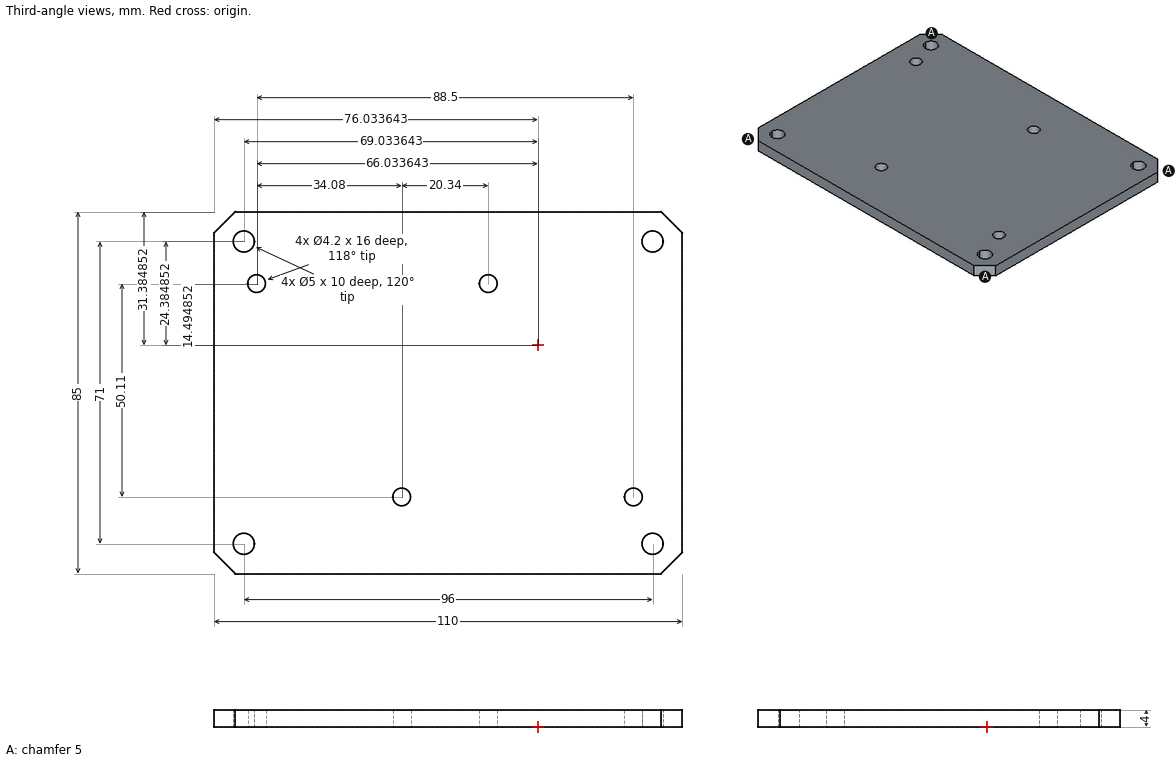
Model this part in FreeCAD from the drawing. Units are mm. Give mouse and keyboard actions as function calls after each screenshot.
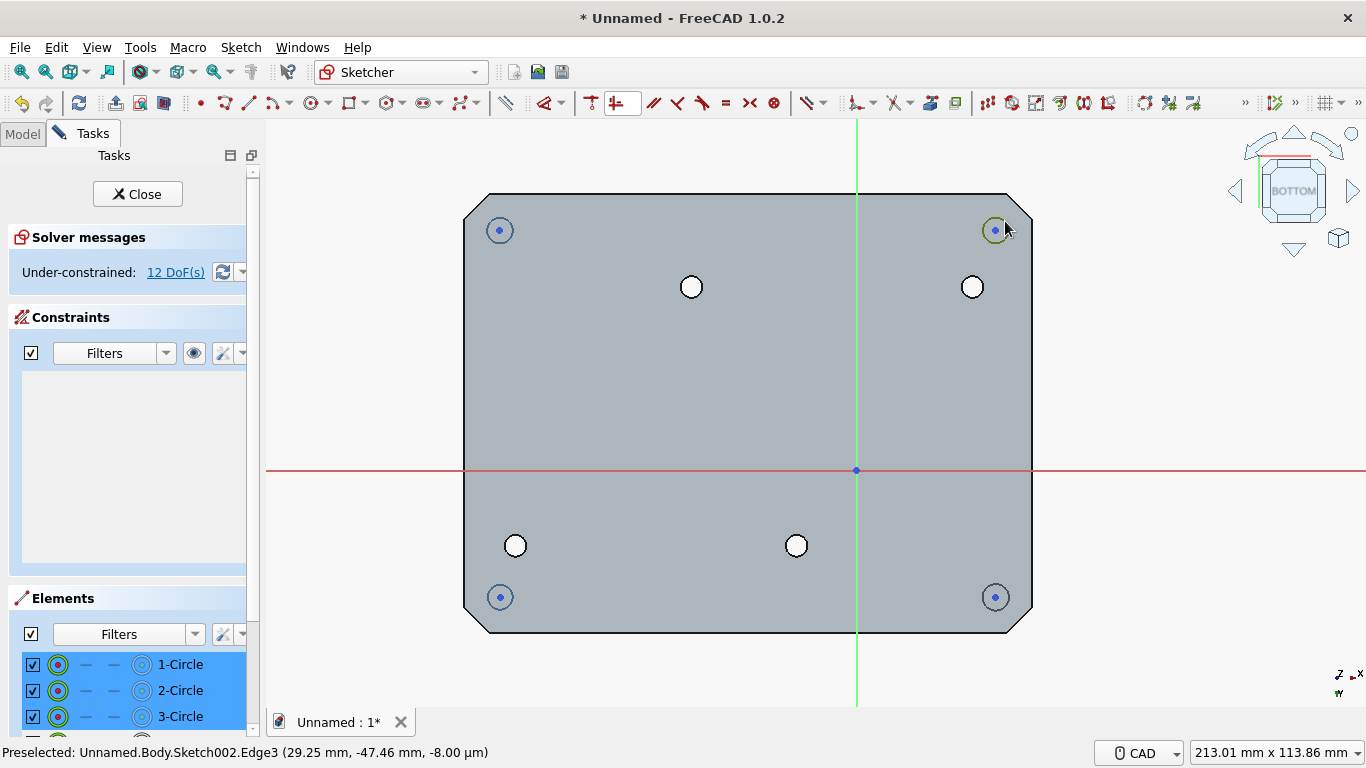
click(1005, 588)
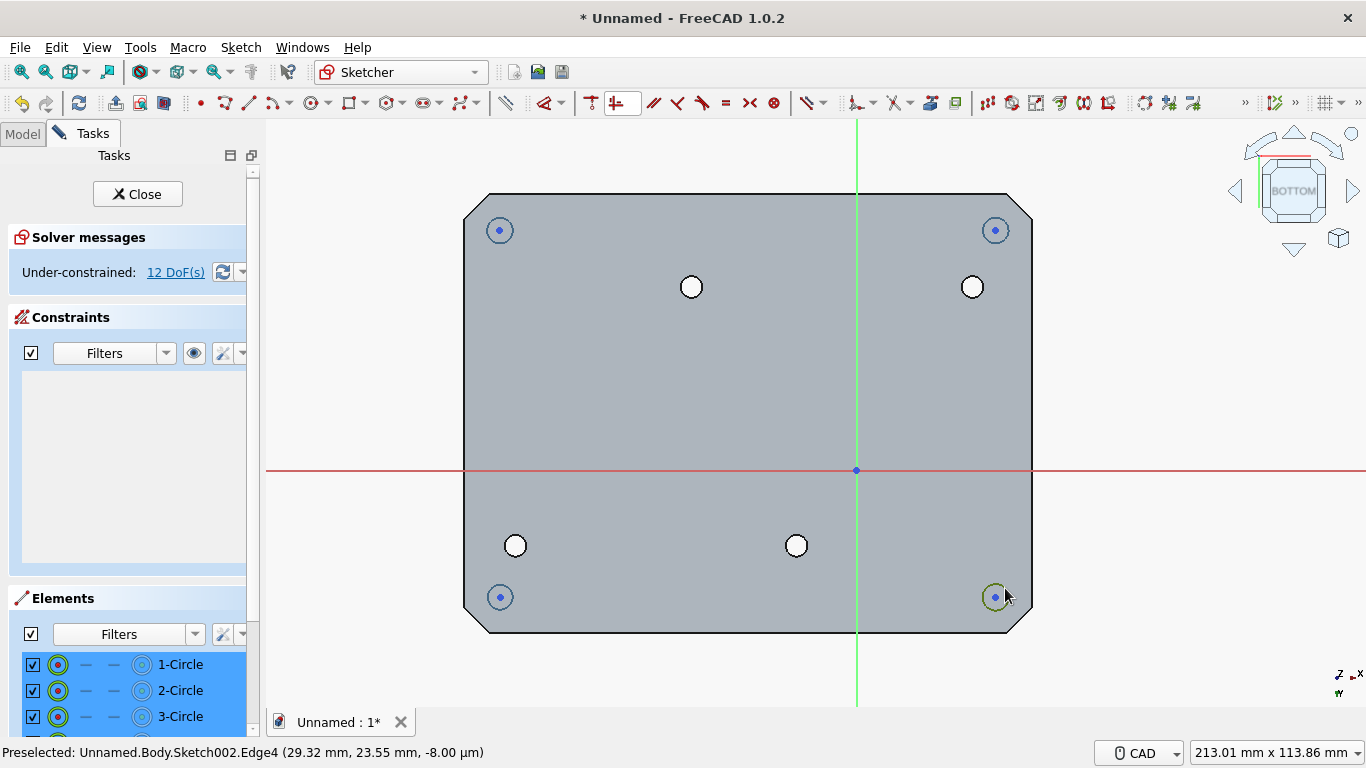
click(726, 104)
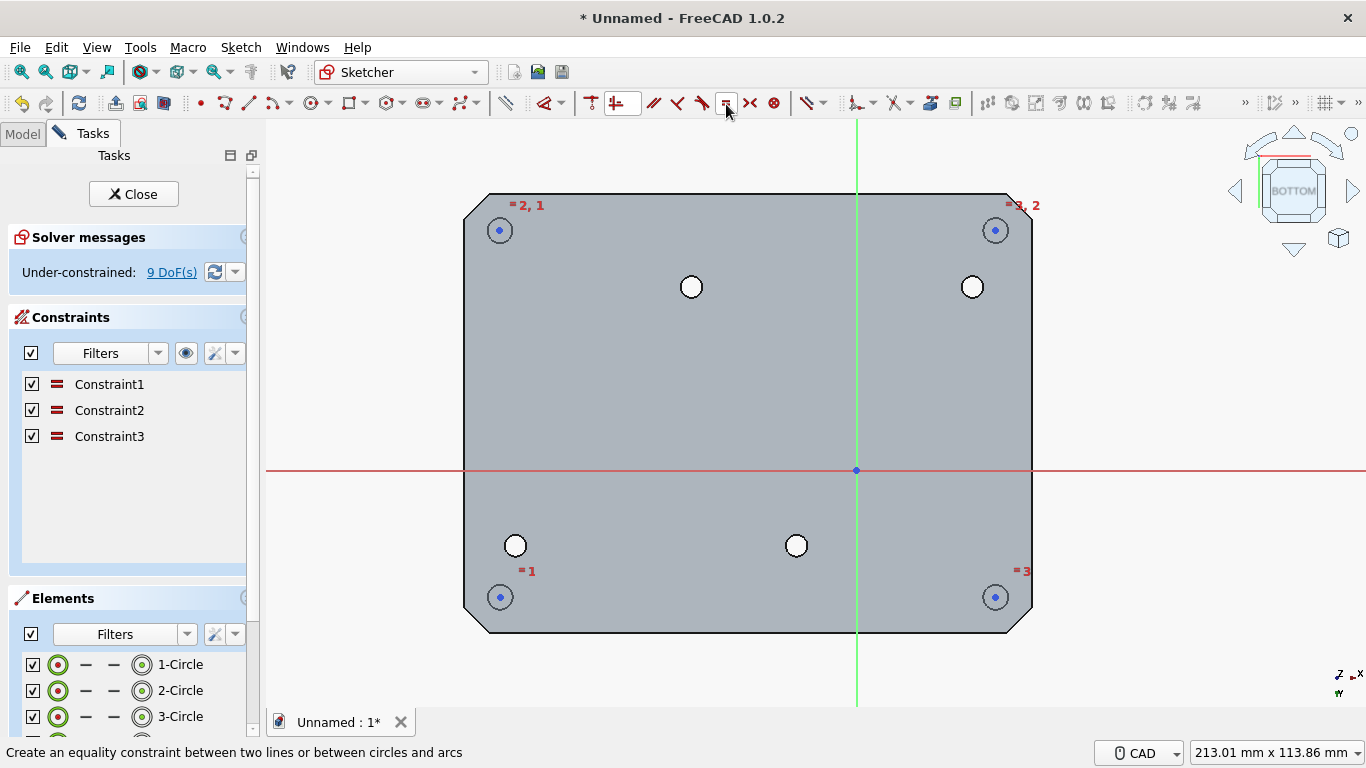
click(500, 597)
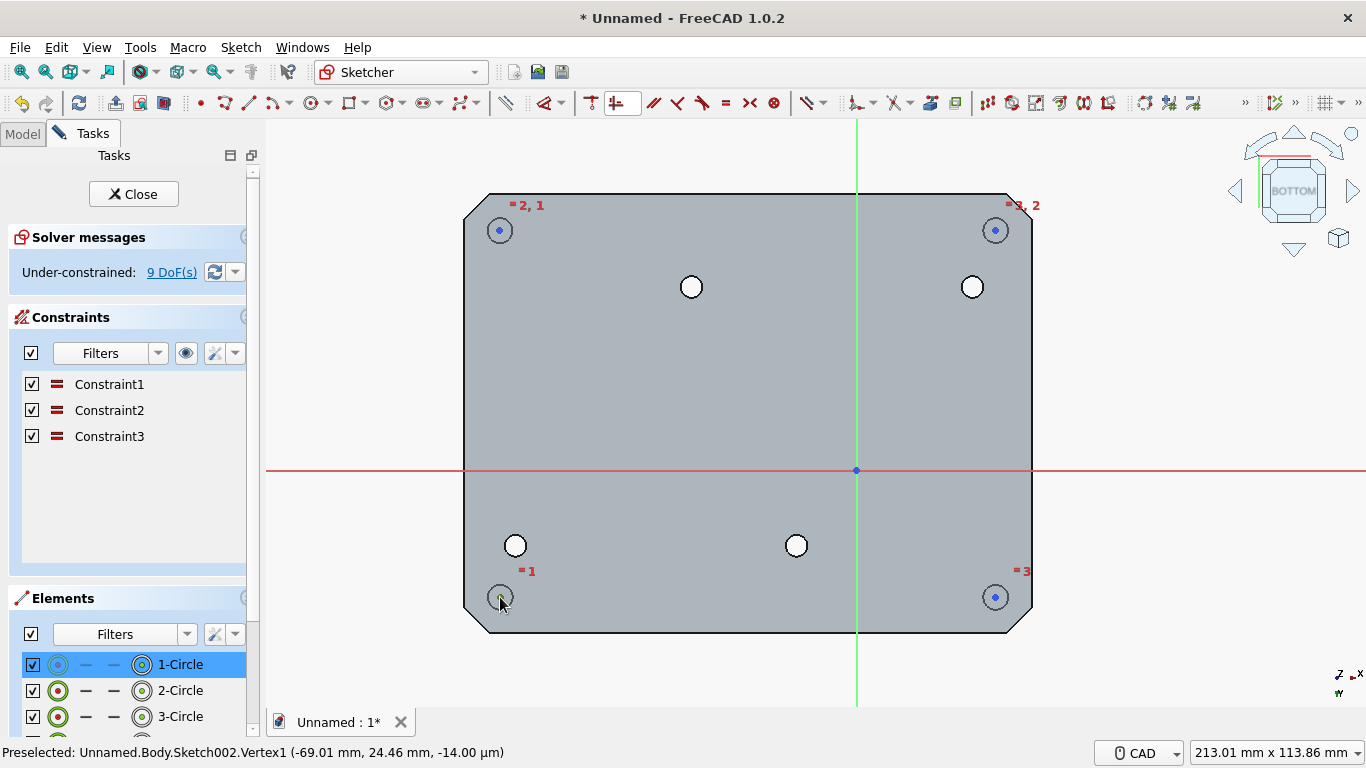
click(500, 231)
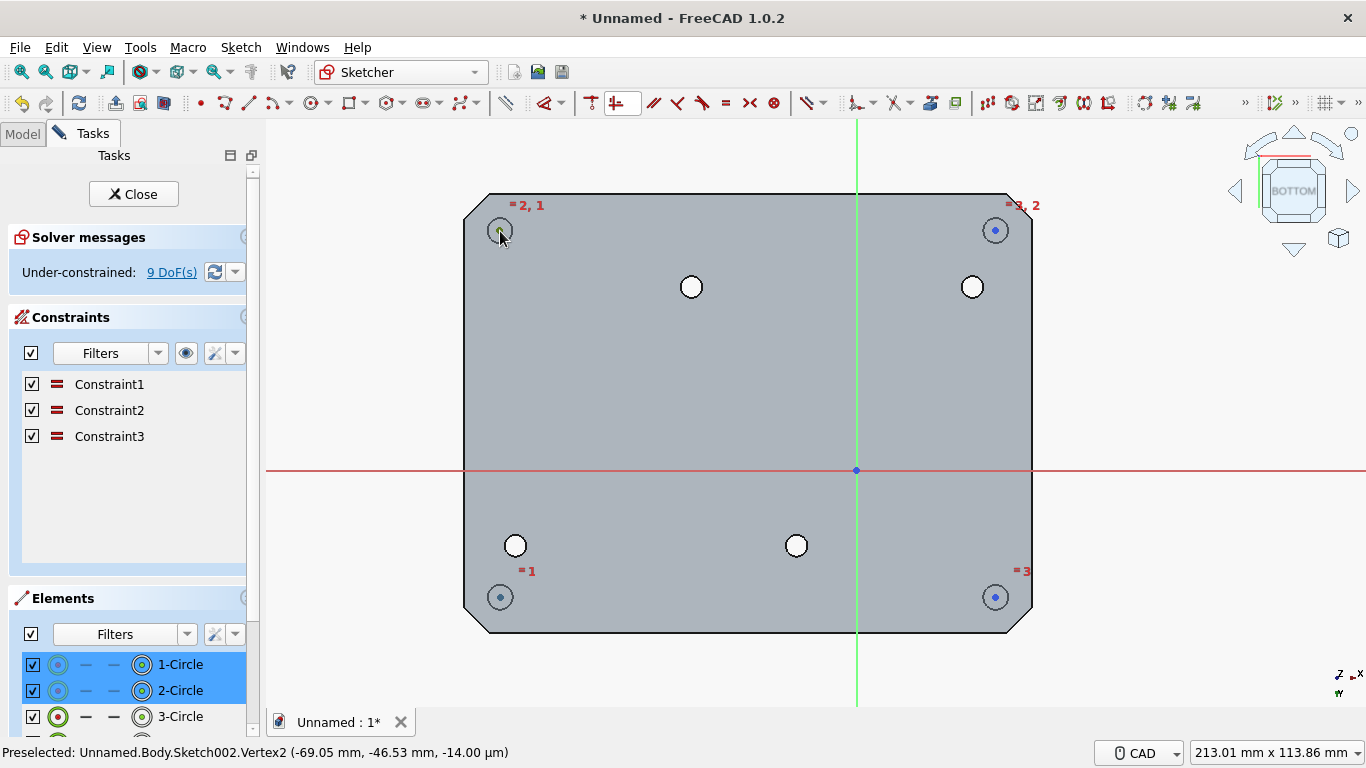
key(v)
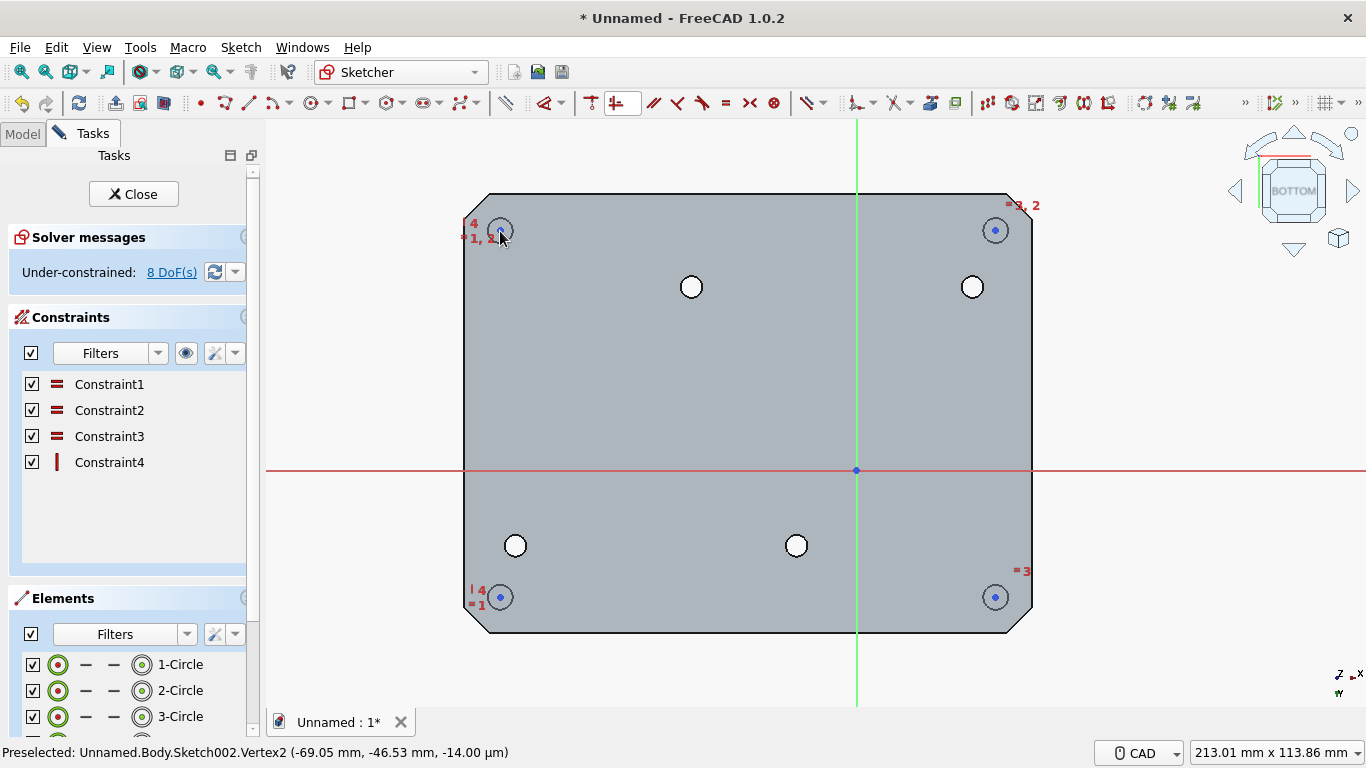
click(500, 231)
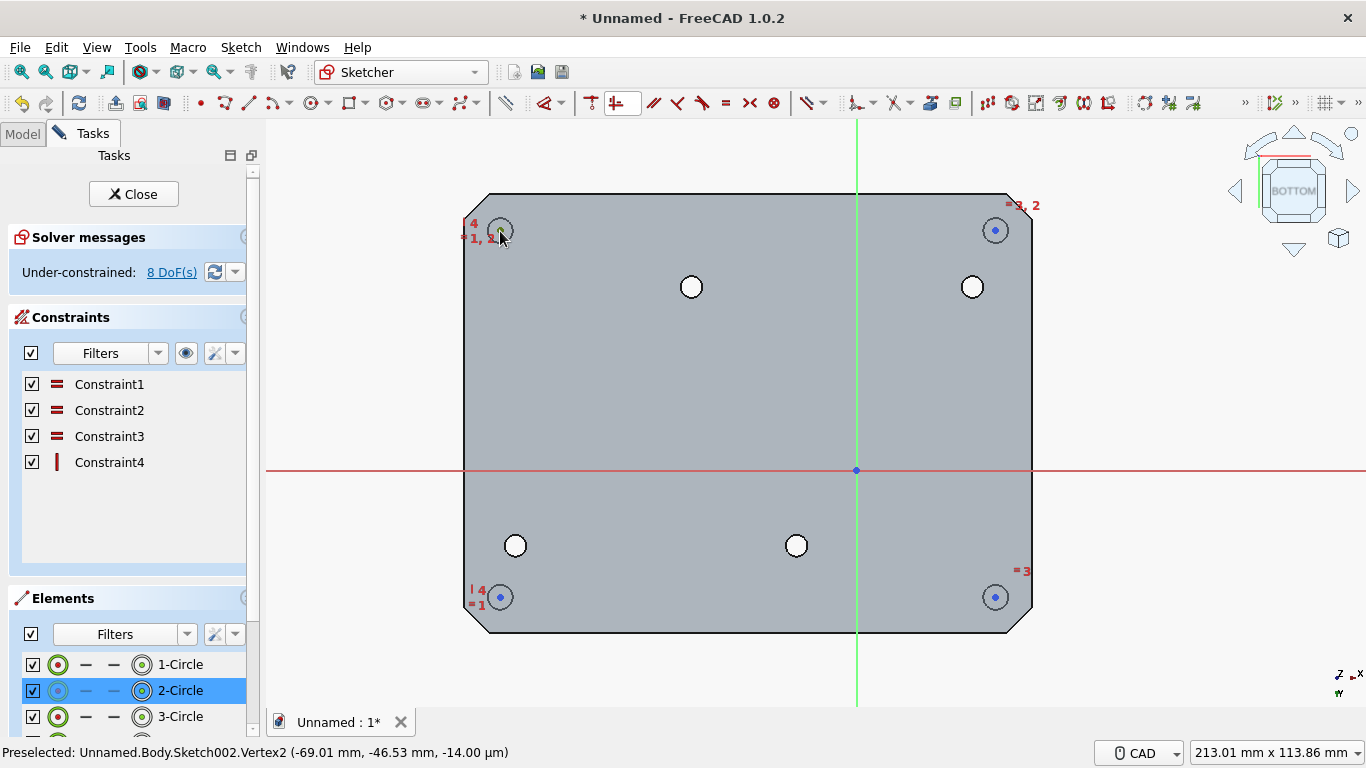
click(996, 231)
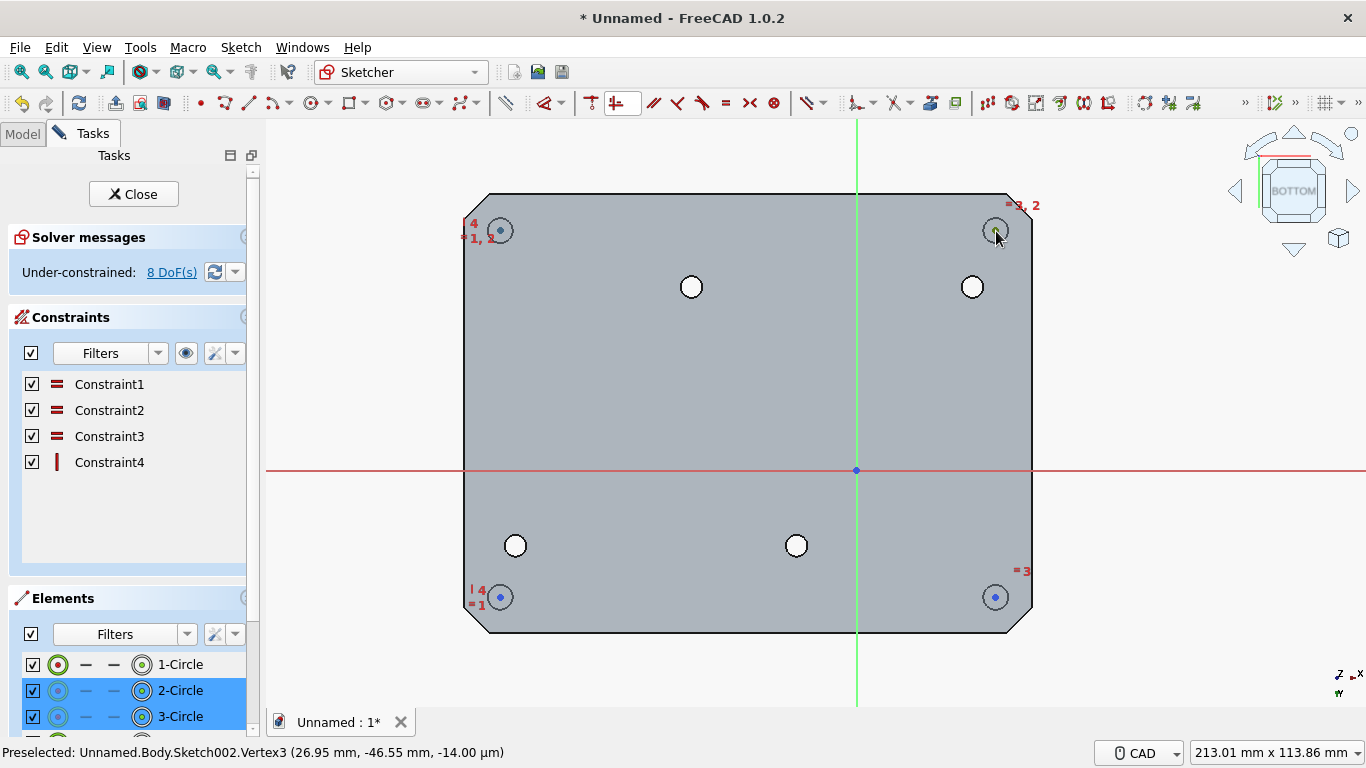
key(h)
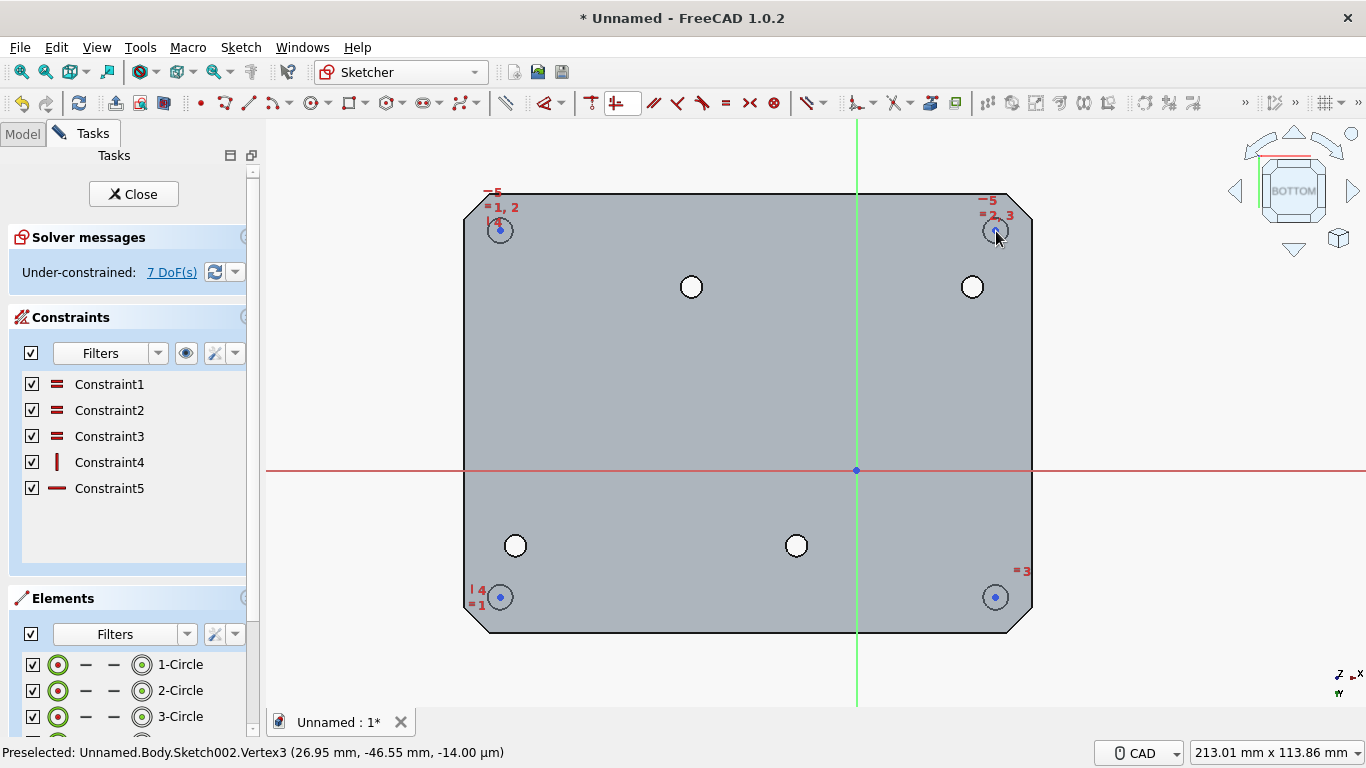
click(996, 231)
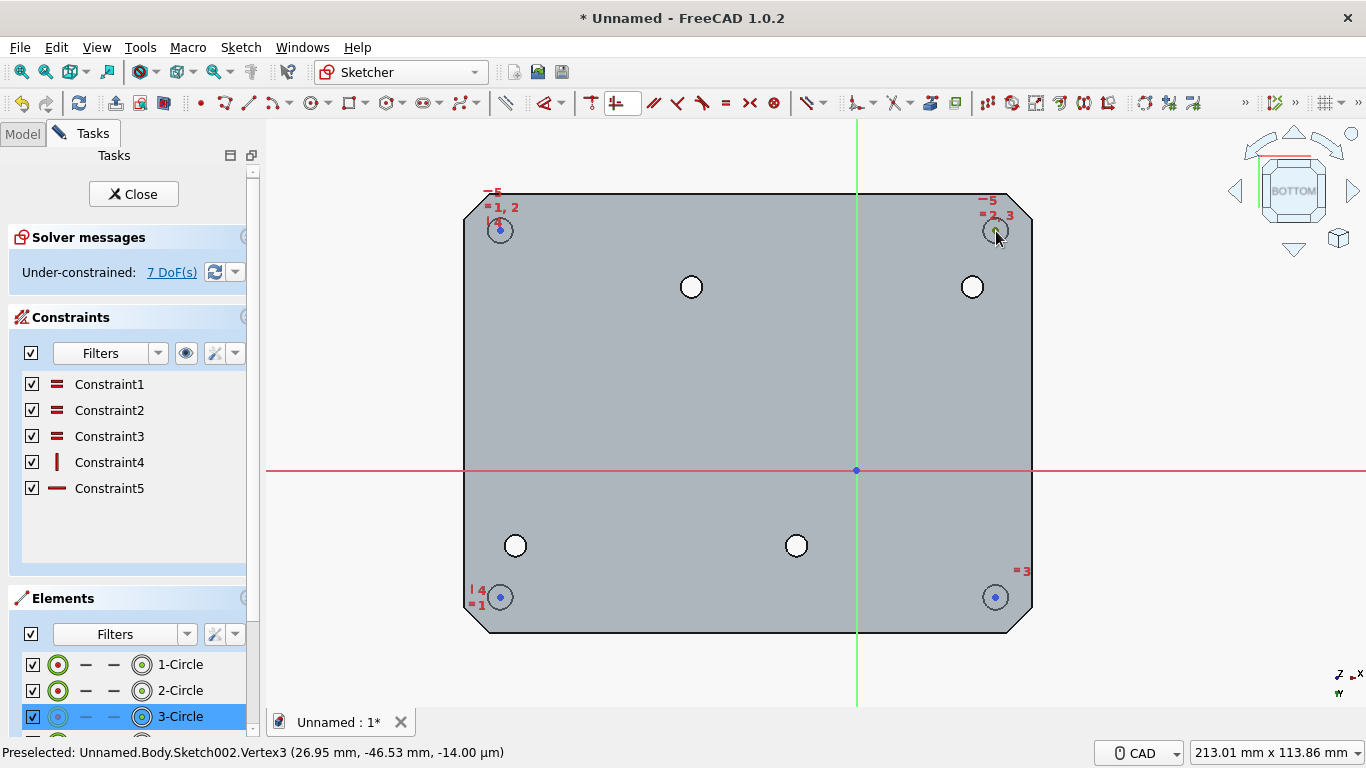
click(996, 597)